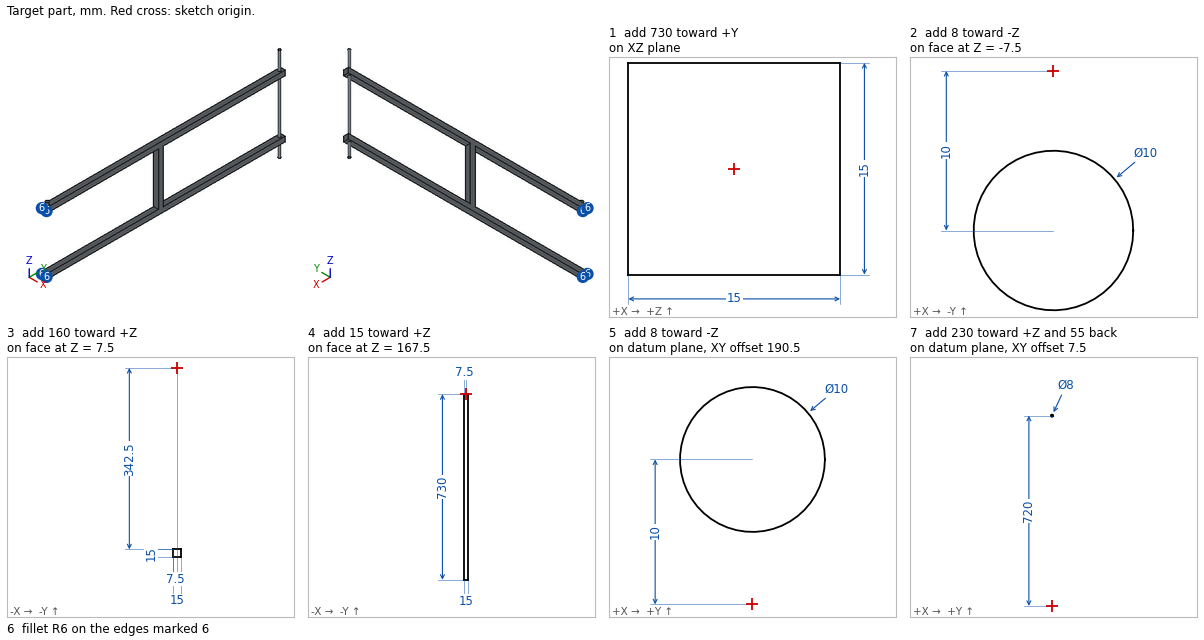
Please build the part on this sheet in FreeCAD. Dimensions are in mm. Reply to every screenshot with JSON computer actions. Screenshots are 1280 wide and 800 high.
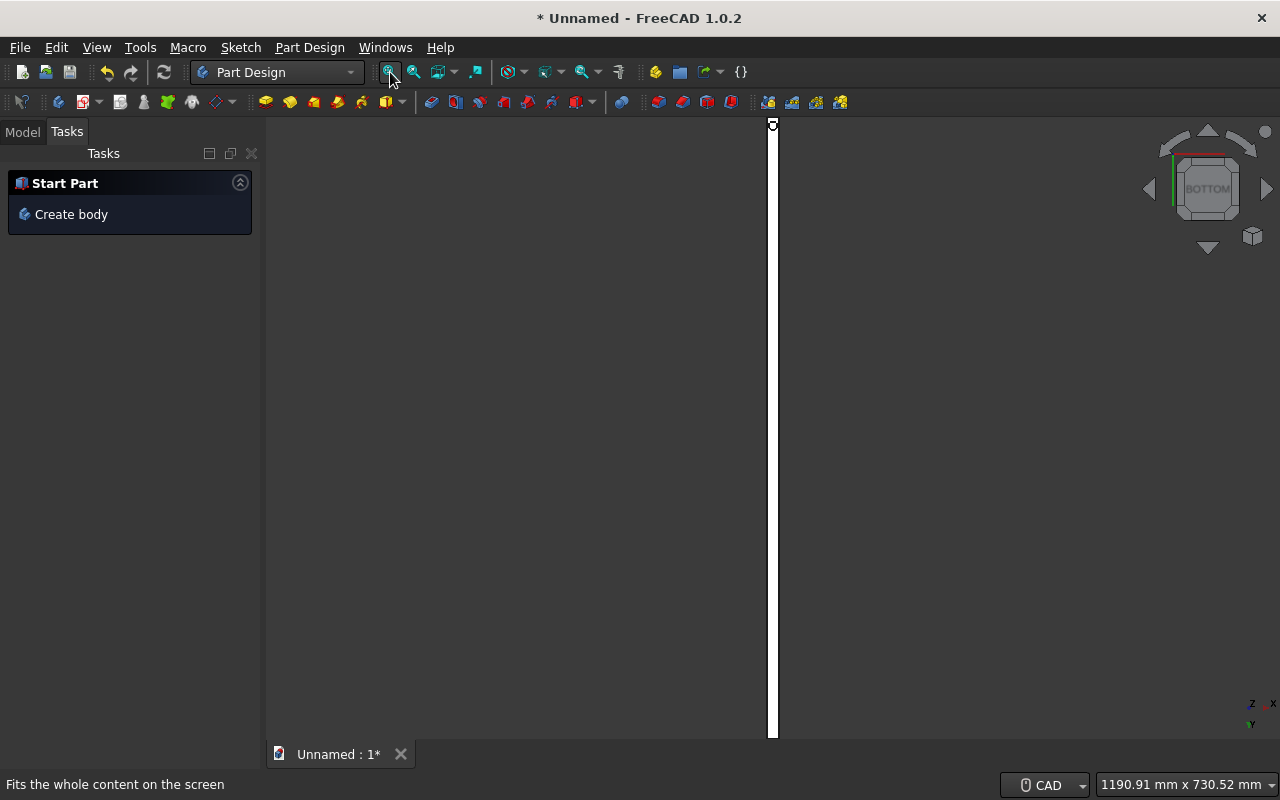
{"action": "key", "text": "0"}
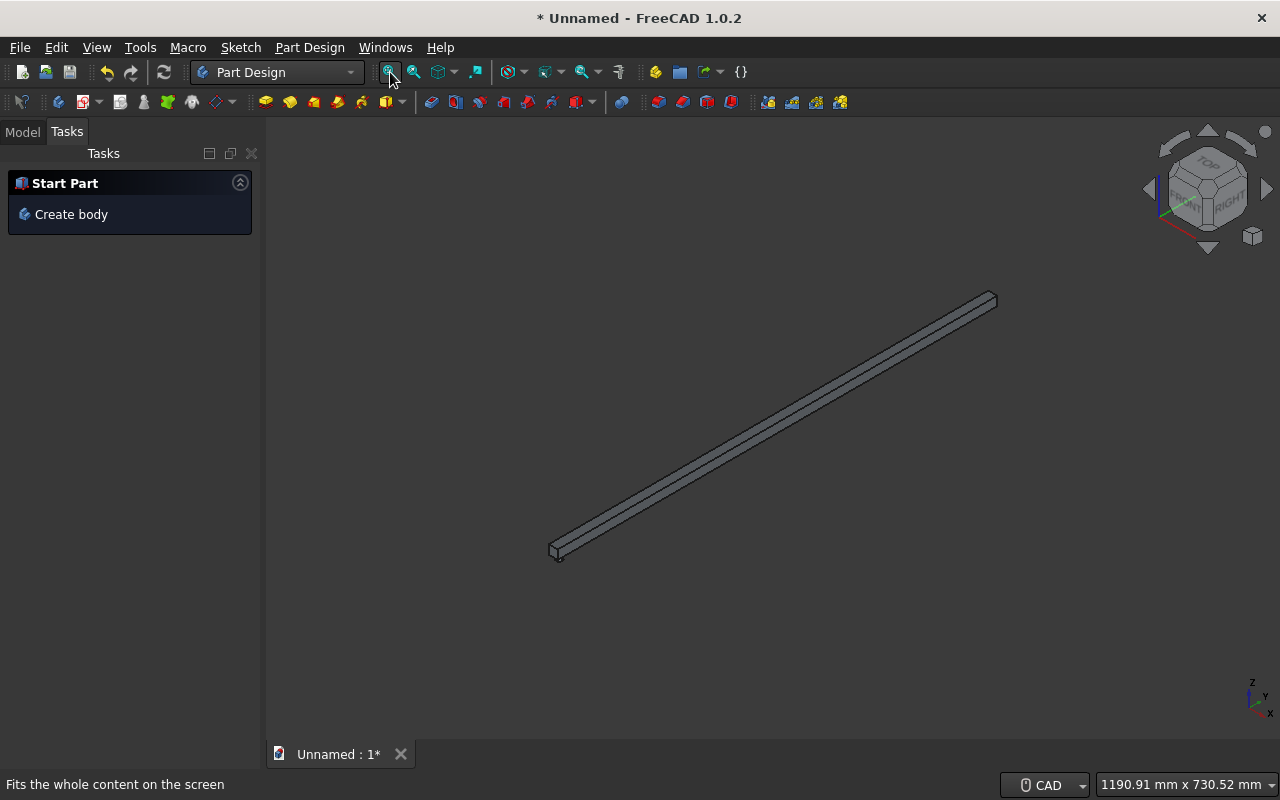
{"action": "left_click", "coordinate": [390, 72]}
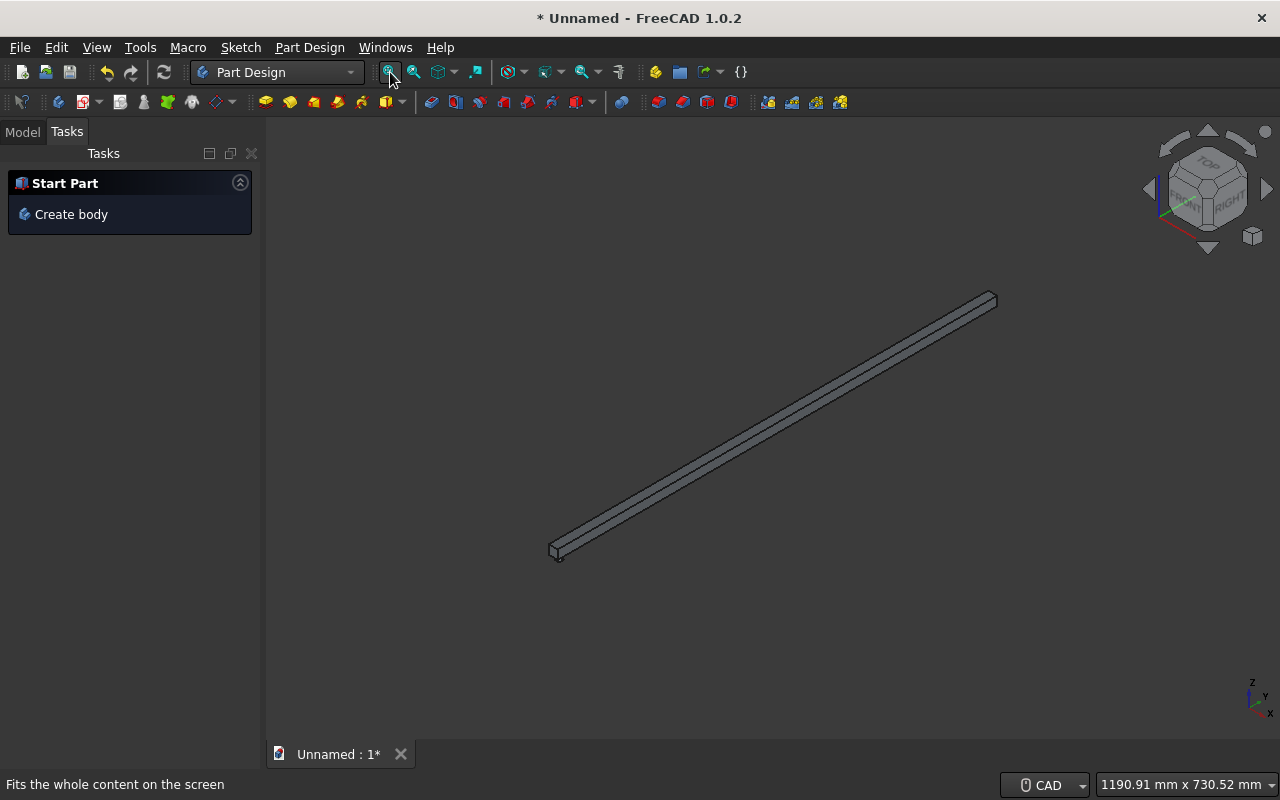
{"action": "scroll", "coordinate": [961, 310], "scroll_direction": "up", "scroll_amount": 4}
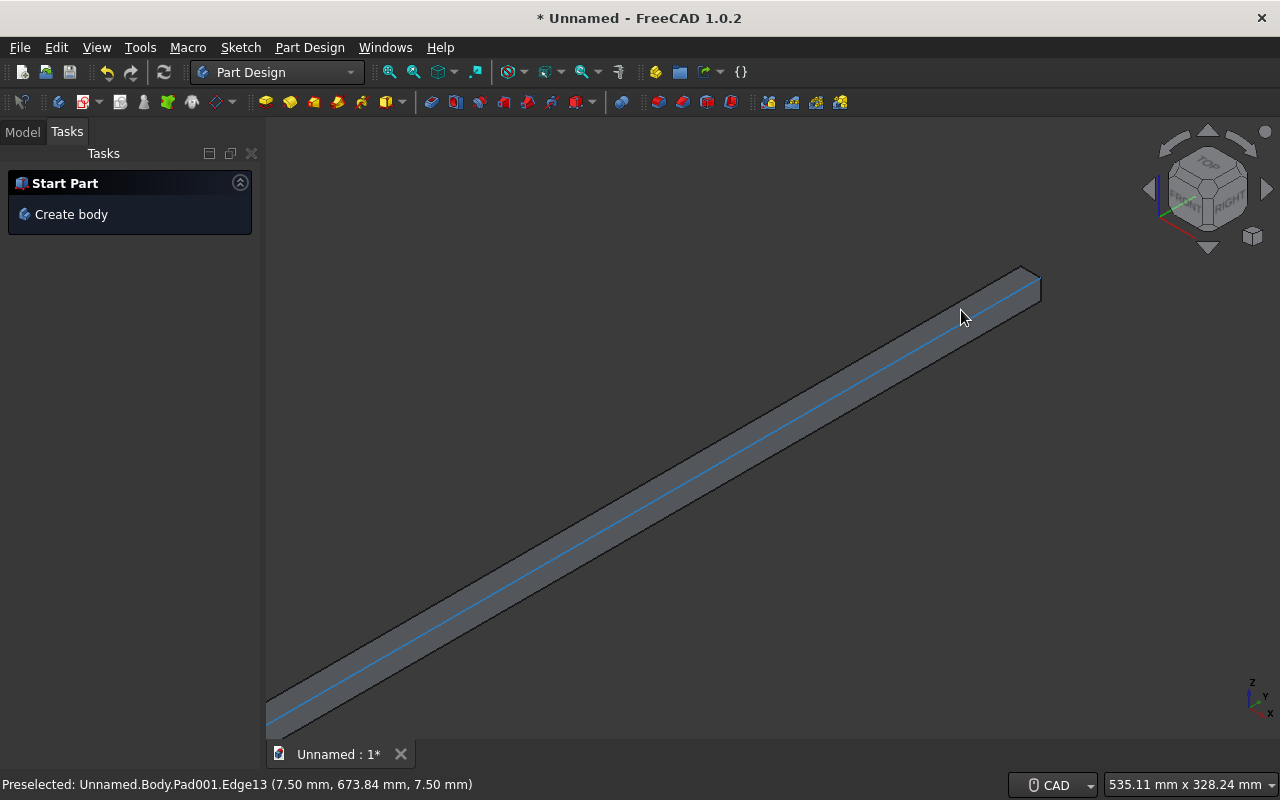
{"action": "left_click", "coordinate": [961, 311]}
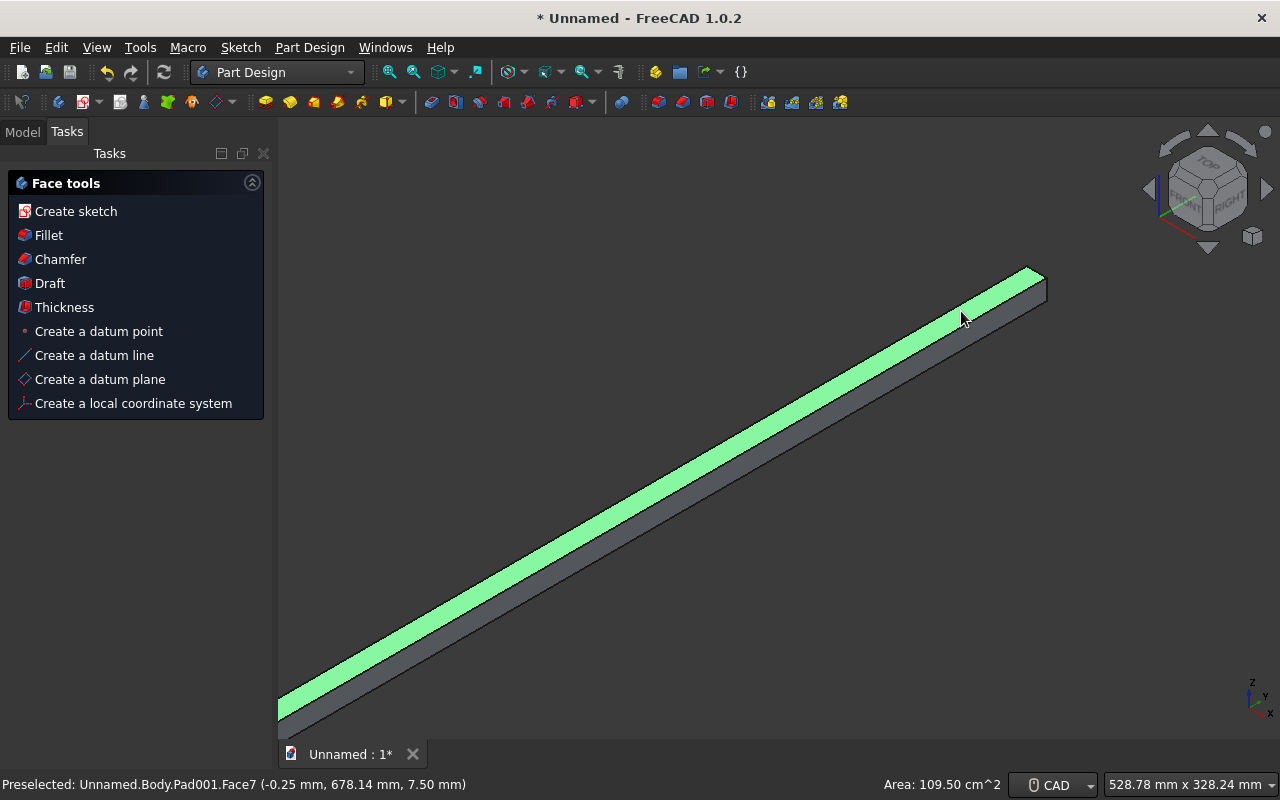
{"action": "left_click", "coordinate": [84, 102]}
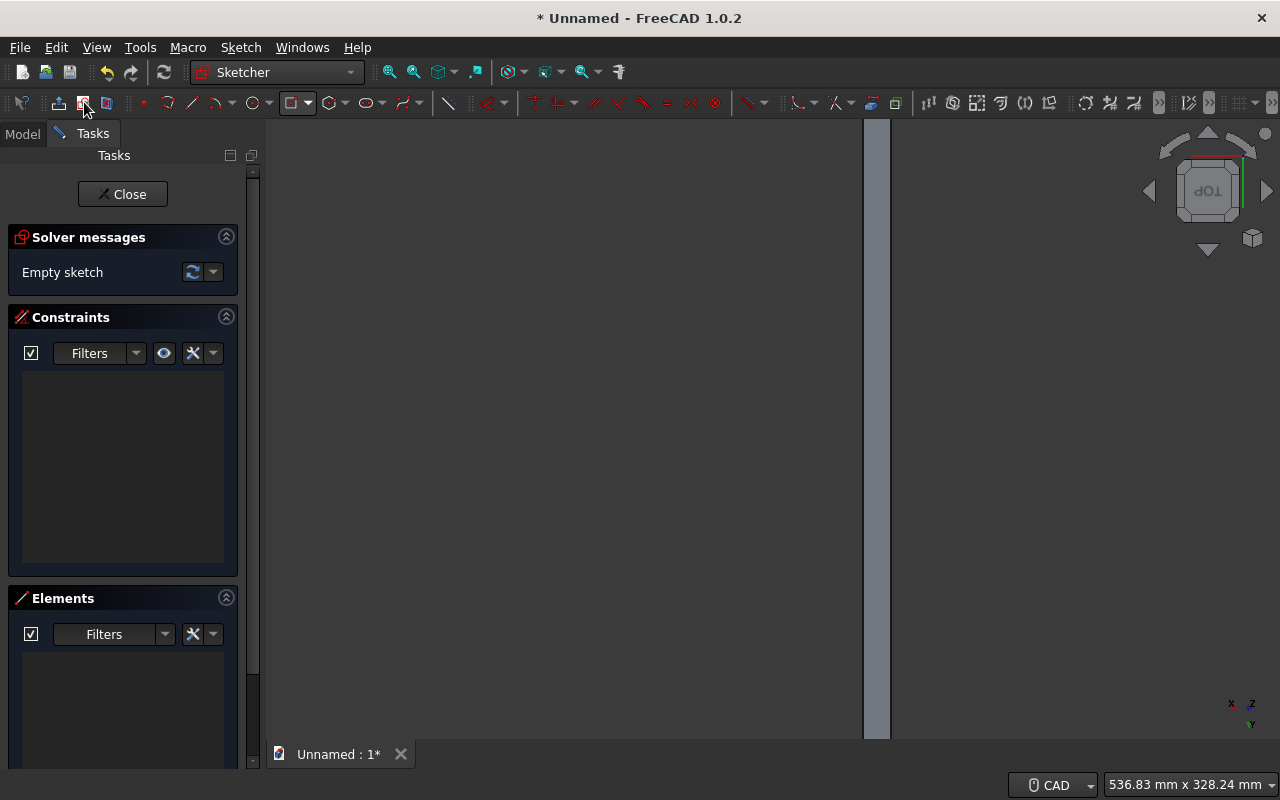
{"action": "scroll", "coordinate": [891, 159], "scroll_direction": "up", "scroll_amount": 13}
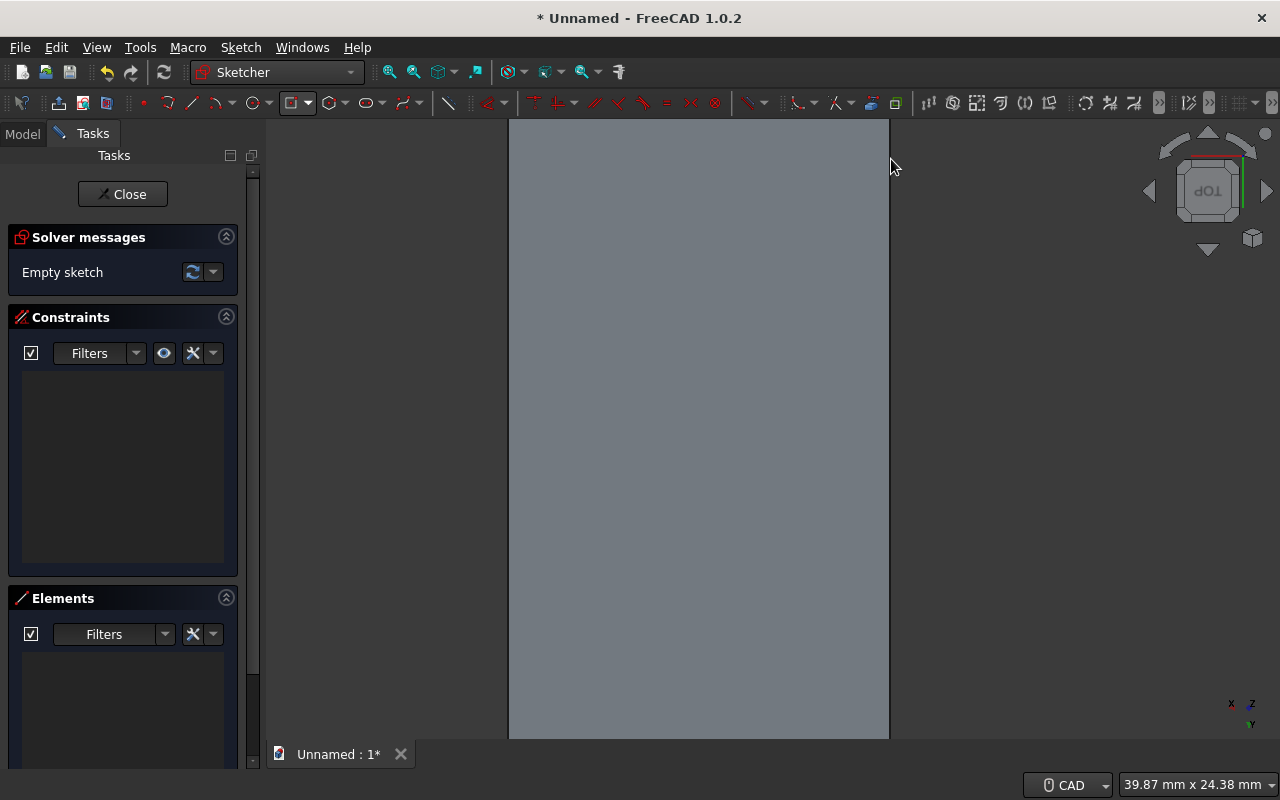
{"action": "left_click", "coordinate": [310, 104]}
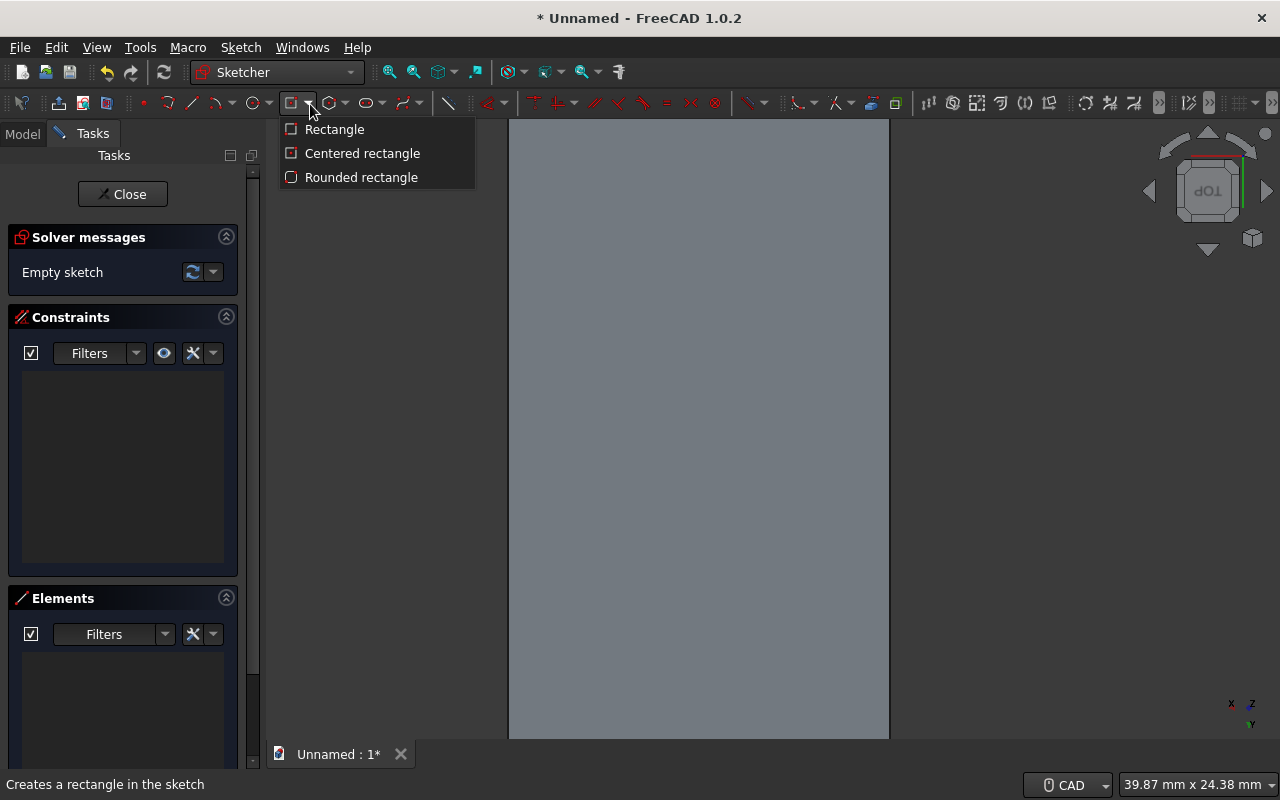
{"action": "left_click", "coordinate": [378, 129]}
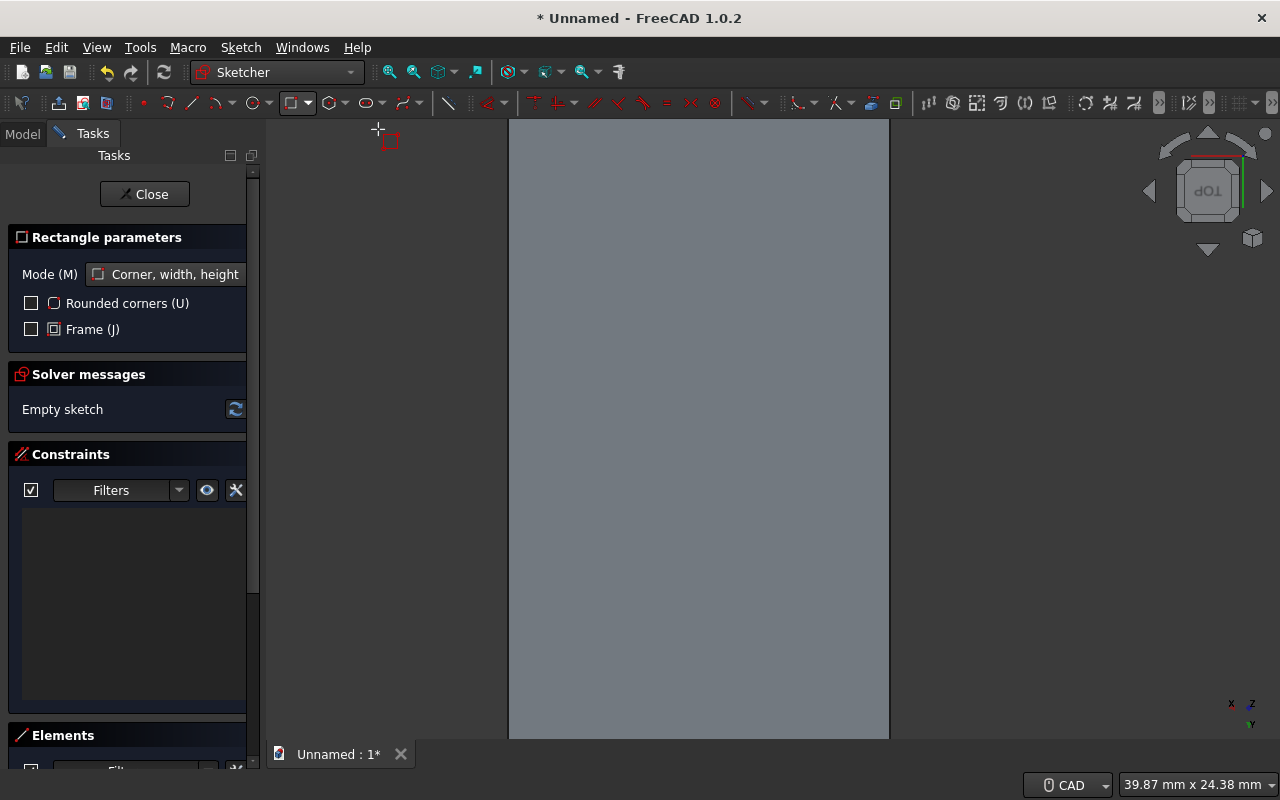
{"action": "left_click", "coordinate": [508, 237]}
{"action": "left_click", "coordinate": [890, 618]}
{"action": "key", "text": "Escape"}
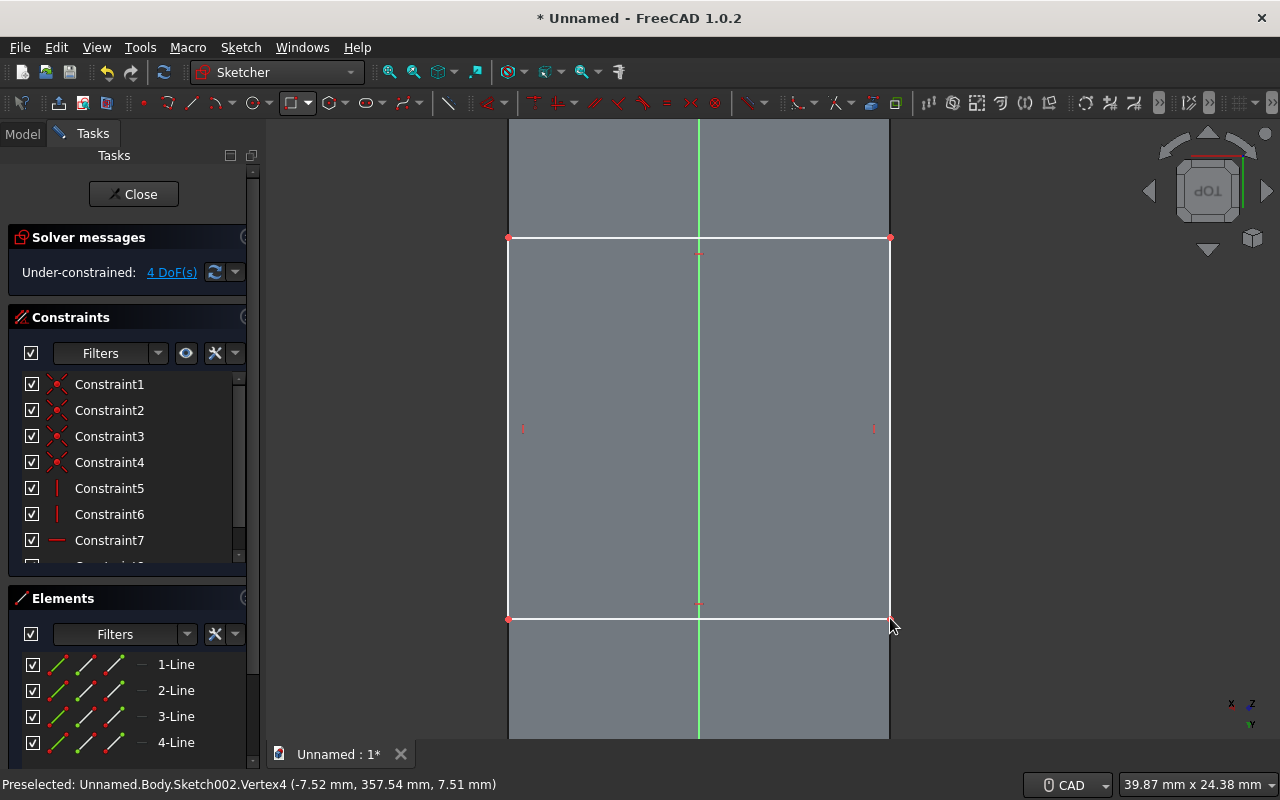
{"action": "left_click", "coordinate": [488, 104]}